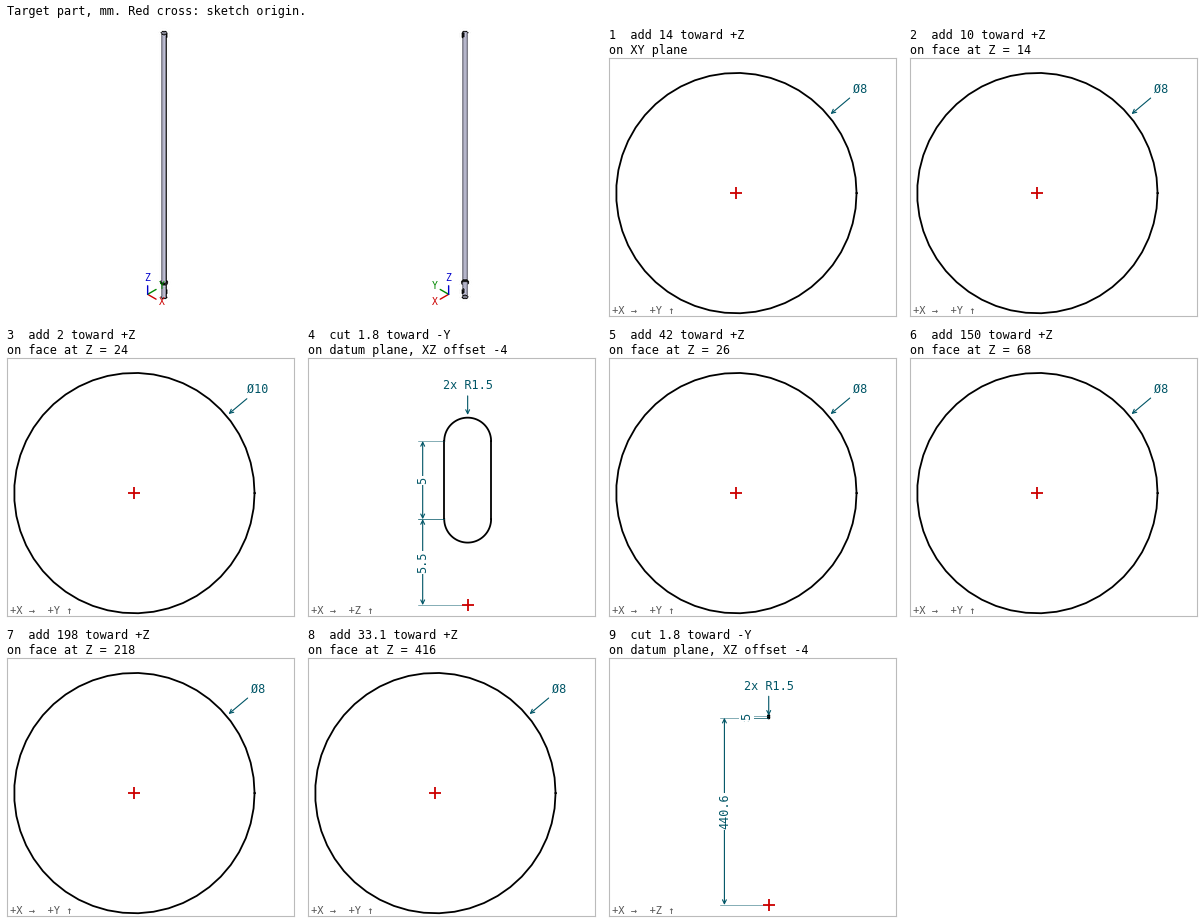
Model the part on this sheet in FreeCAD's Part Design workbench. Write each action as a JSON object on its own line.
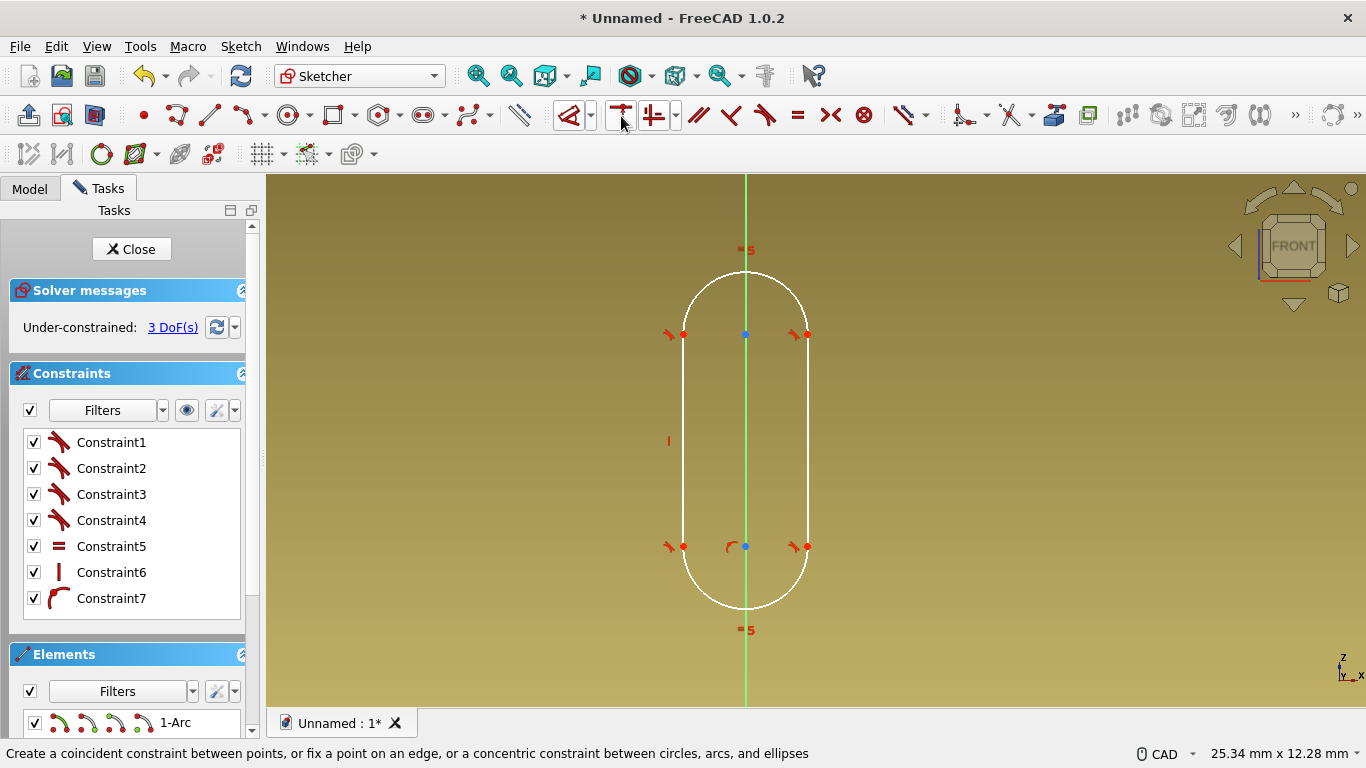
{"action": "left_click", "coordinate": [709, 597]}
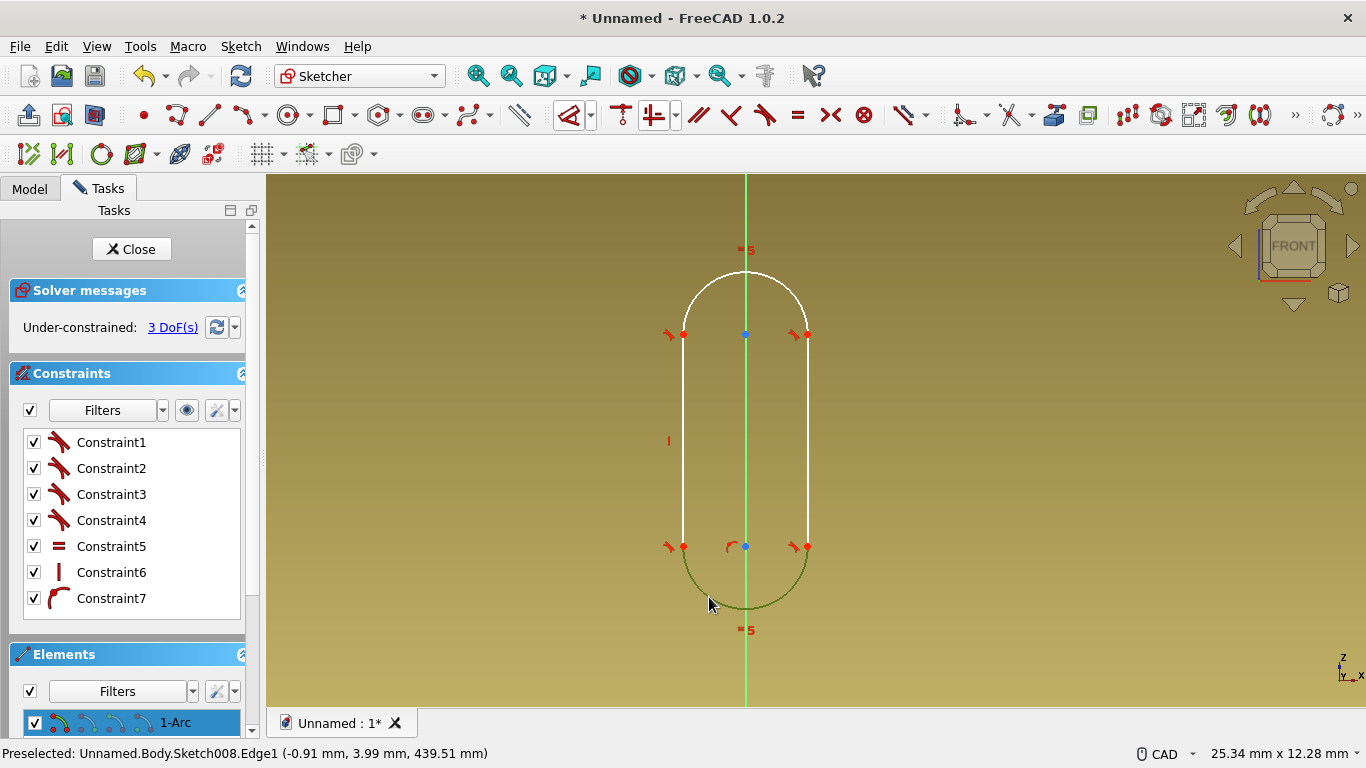
{"action": "key", "text": "k r"}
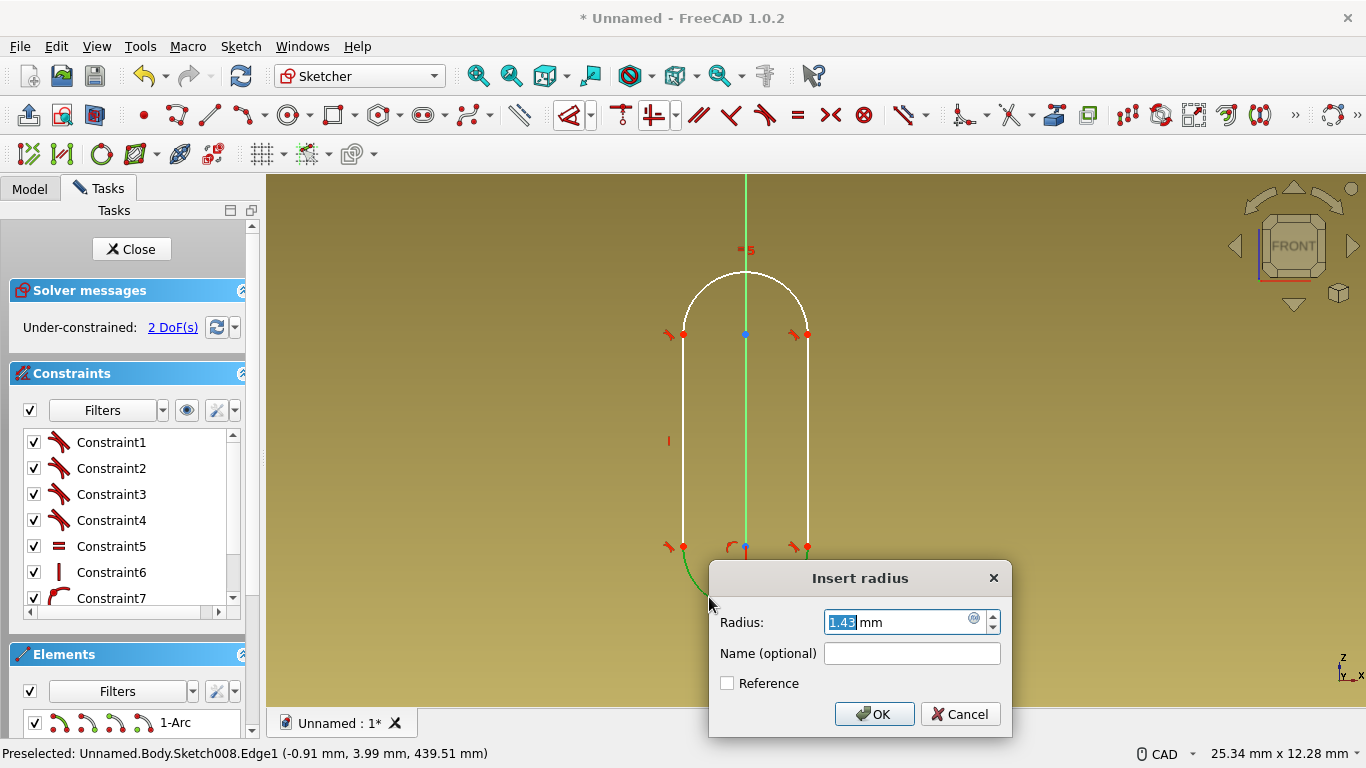
{"action": "type", "text": "1.5"}
{"action": "key", "text": "Return"}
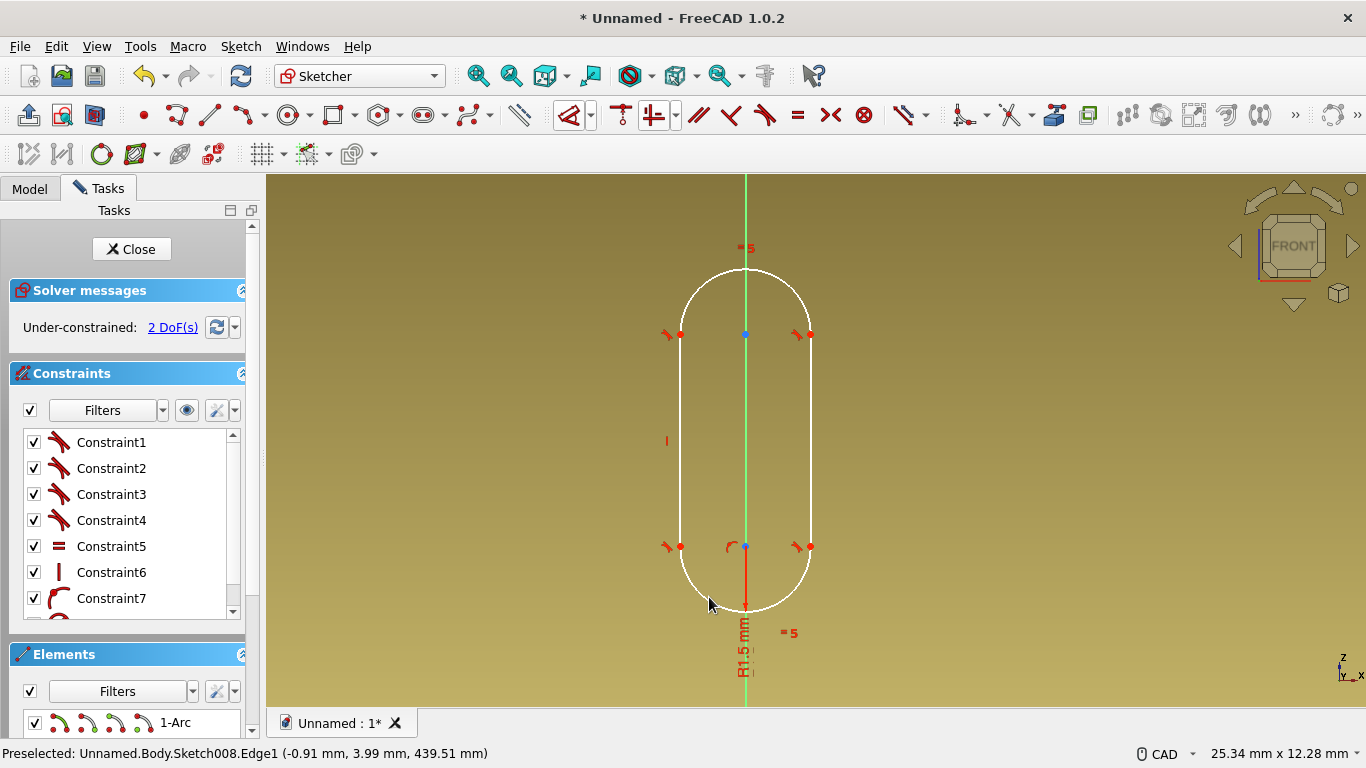
{"action": "left_click", "coordinate": [680, 483]}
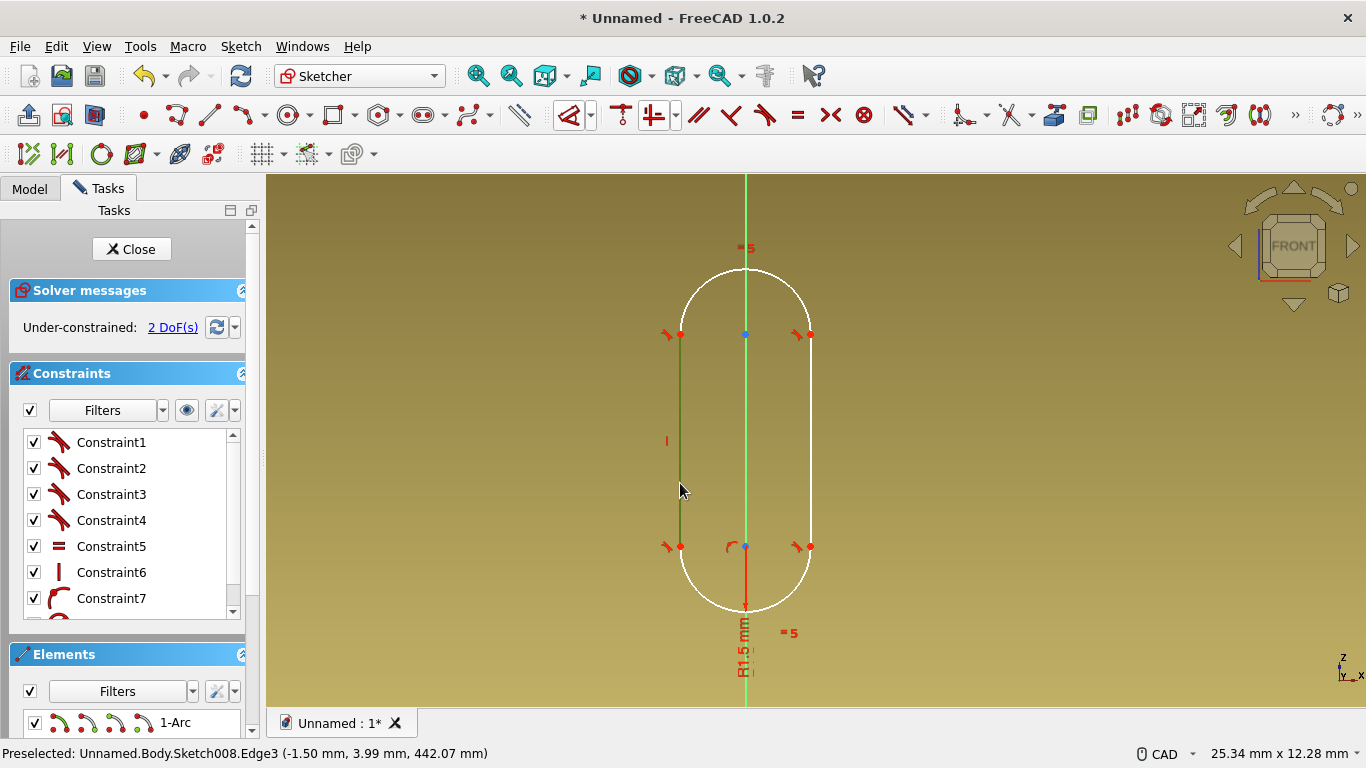
{"action": "left_click", "coordinate": [590, 116]}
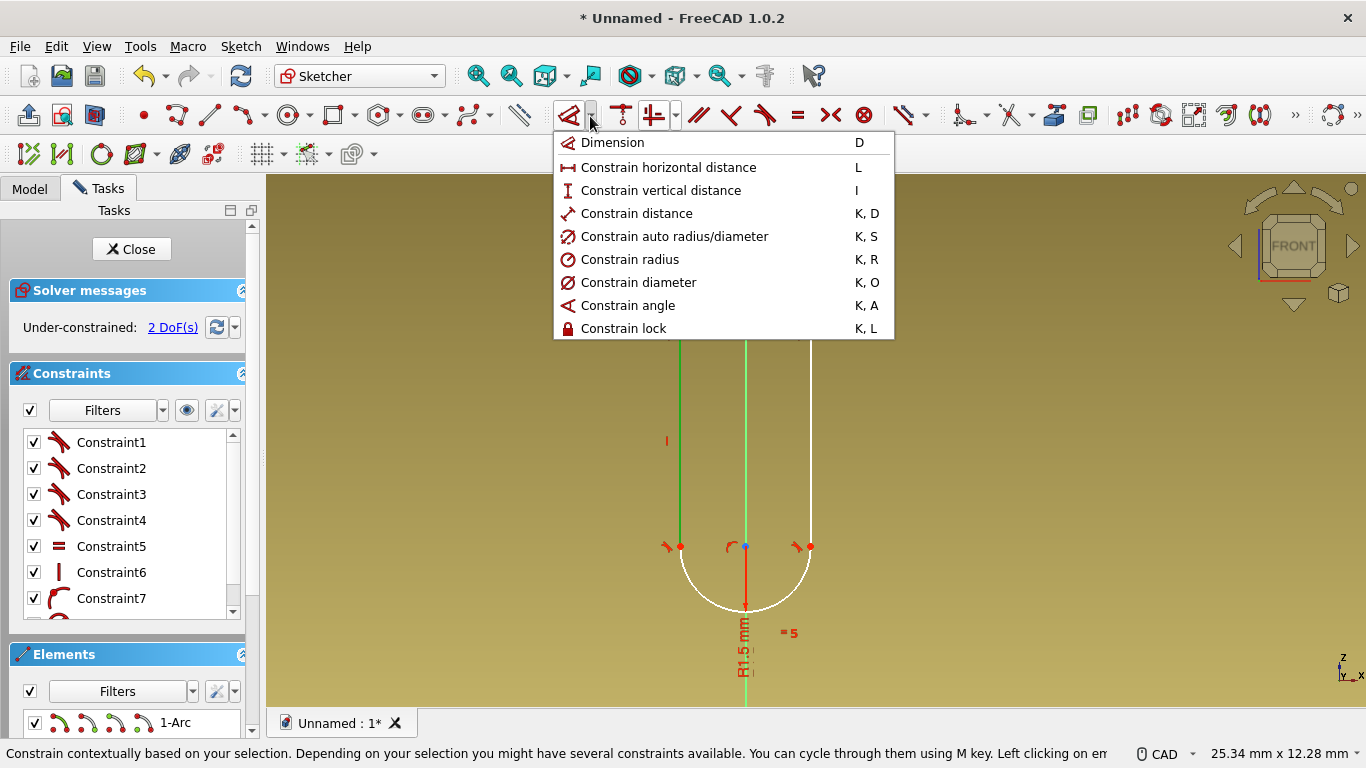
{"action": "left_click", "coordinate": [724, 190]}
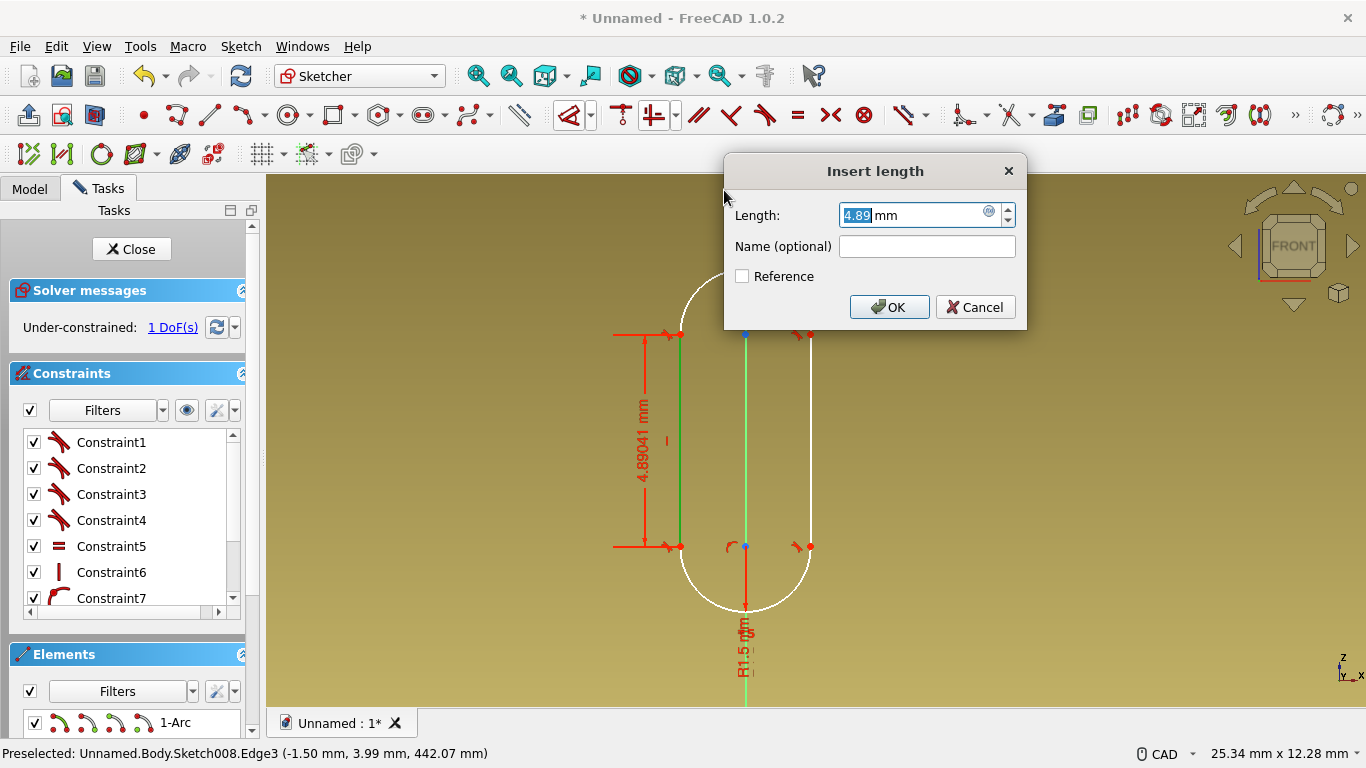
{"action": "type", "text": "5"}
{"action": "key", "text": "Return"}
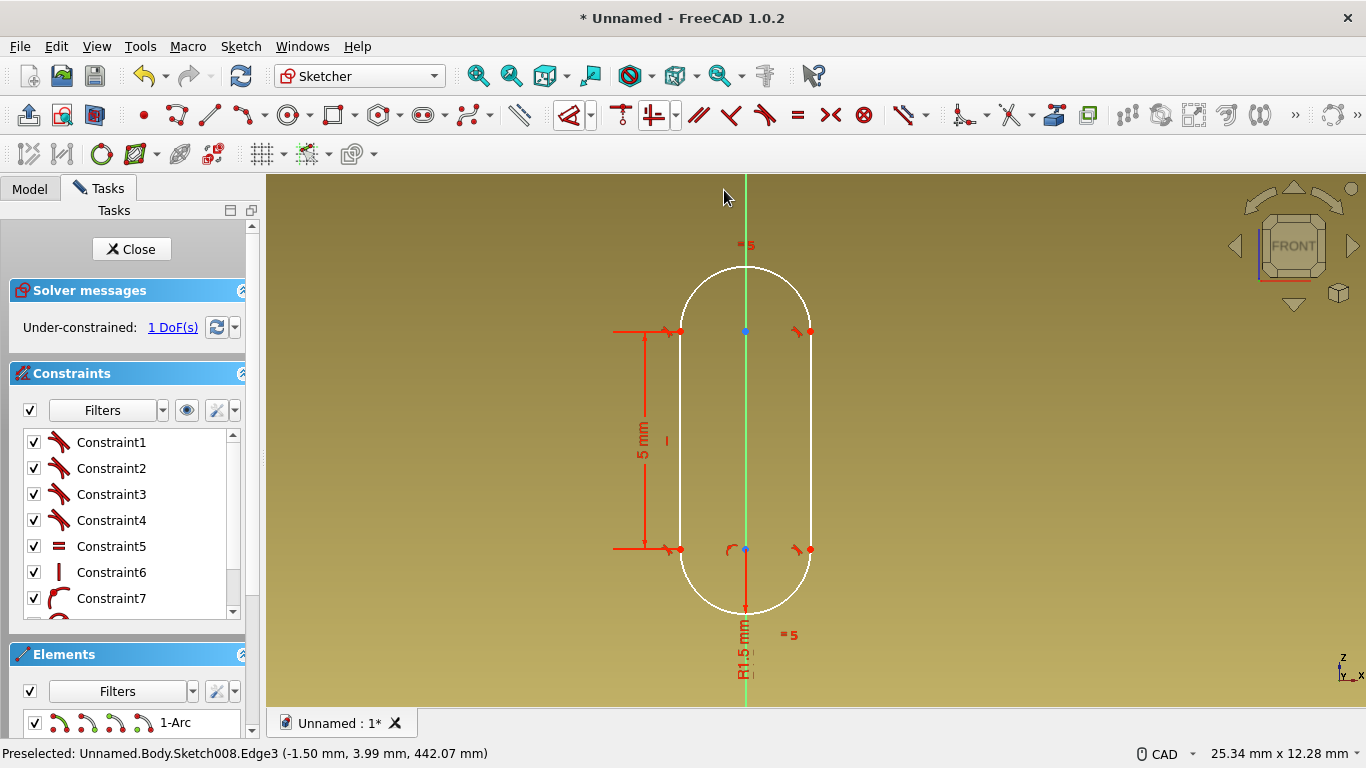
{"action": "left_click", "coordinate": [680, 549]}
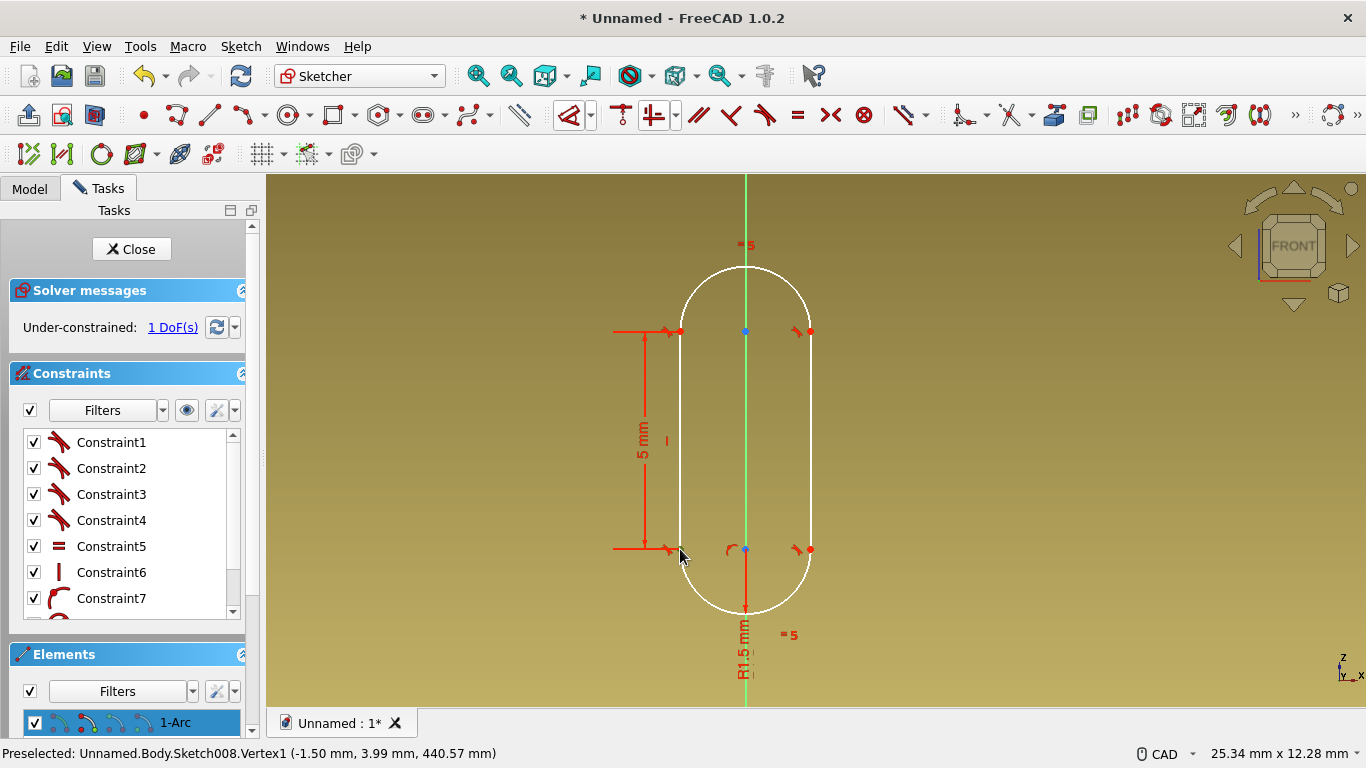
{"action": "left_click", "coordinate": [590, 116]}